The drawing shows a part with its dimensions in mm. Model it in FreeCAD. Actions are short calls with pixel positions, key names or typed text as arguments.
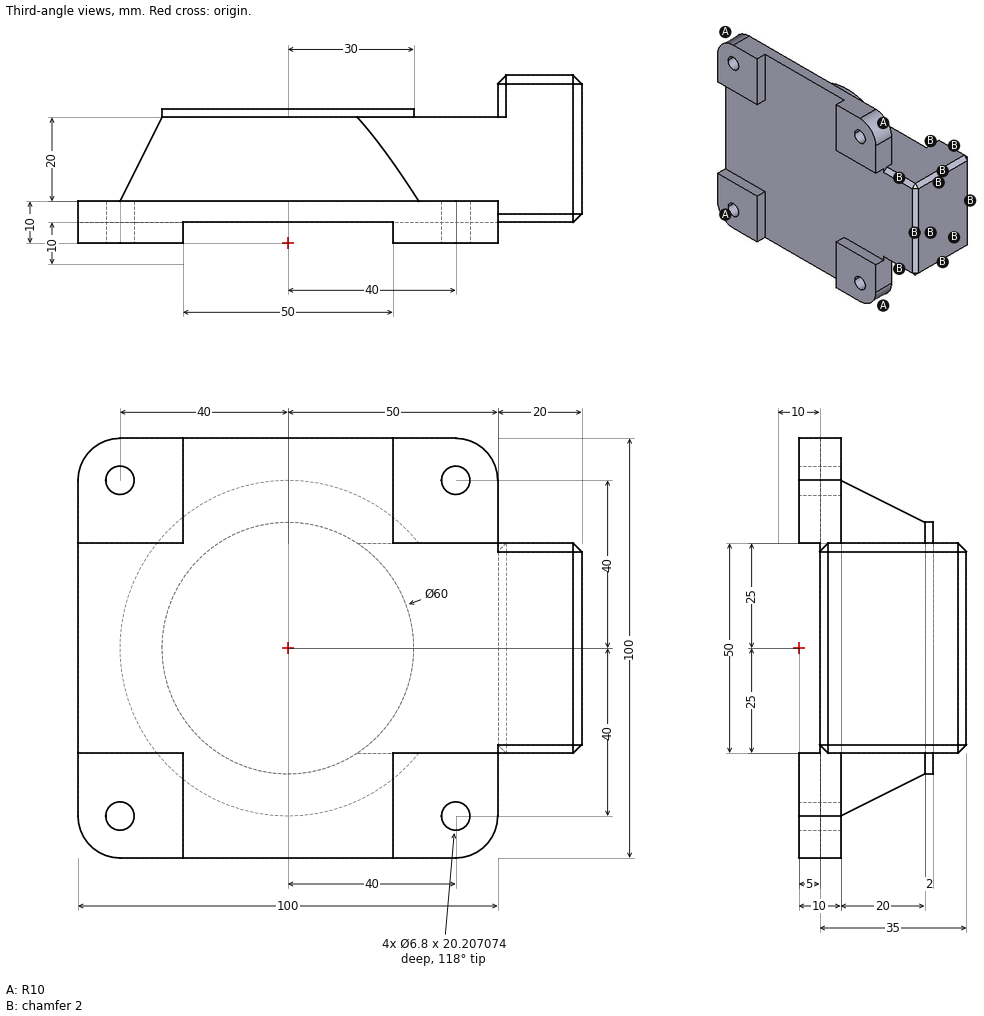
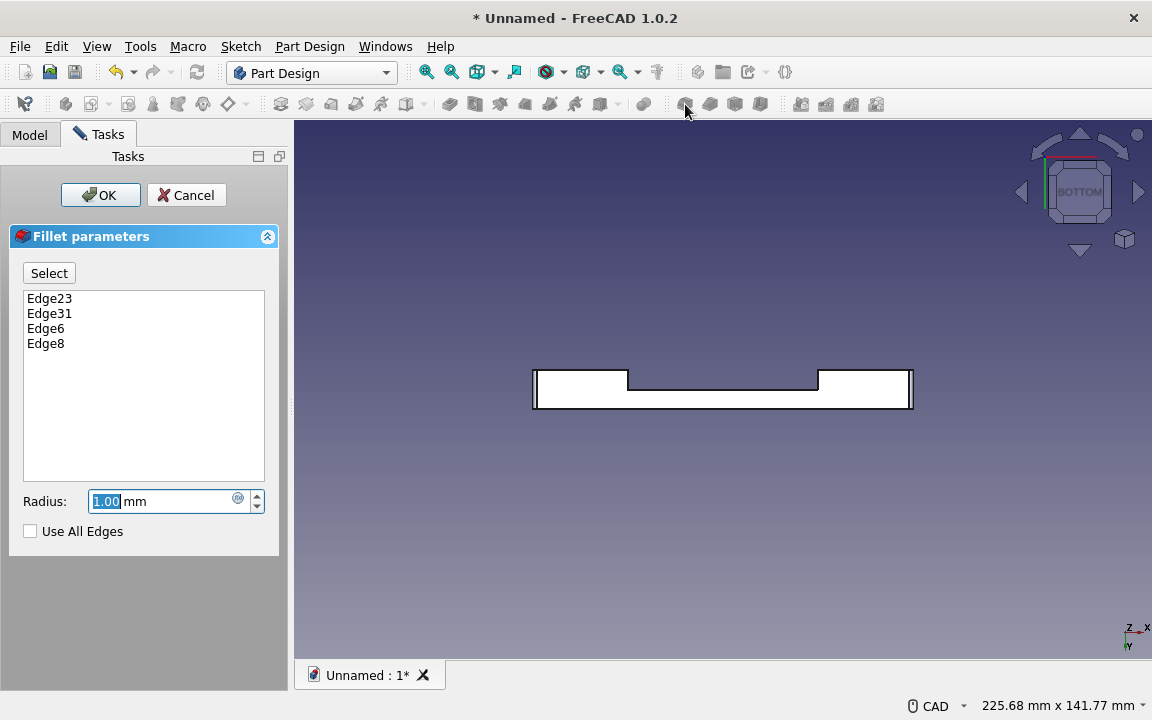
text(10)
key(Tab)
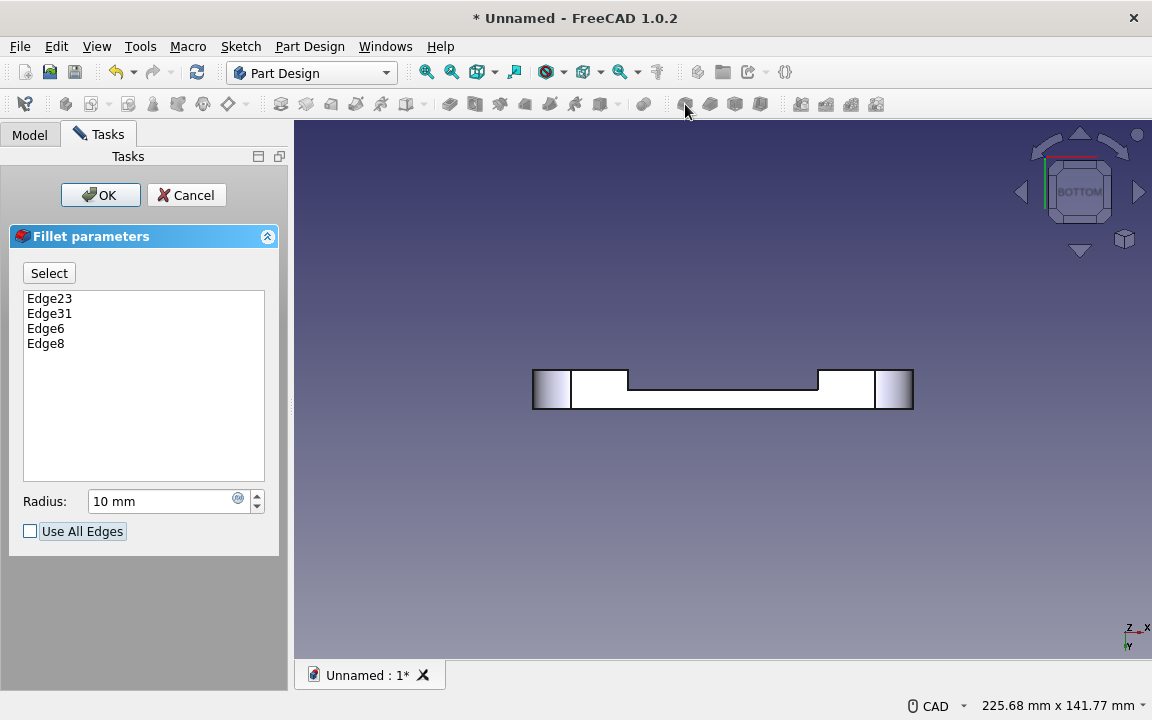
click(101, 195)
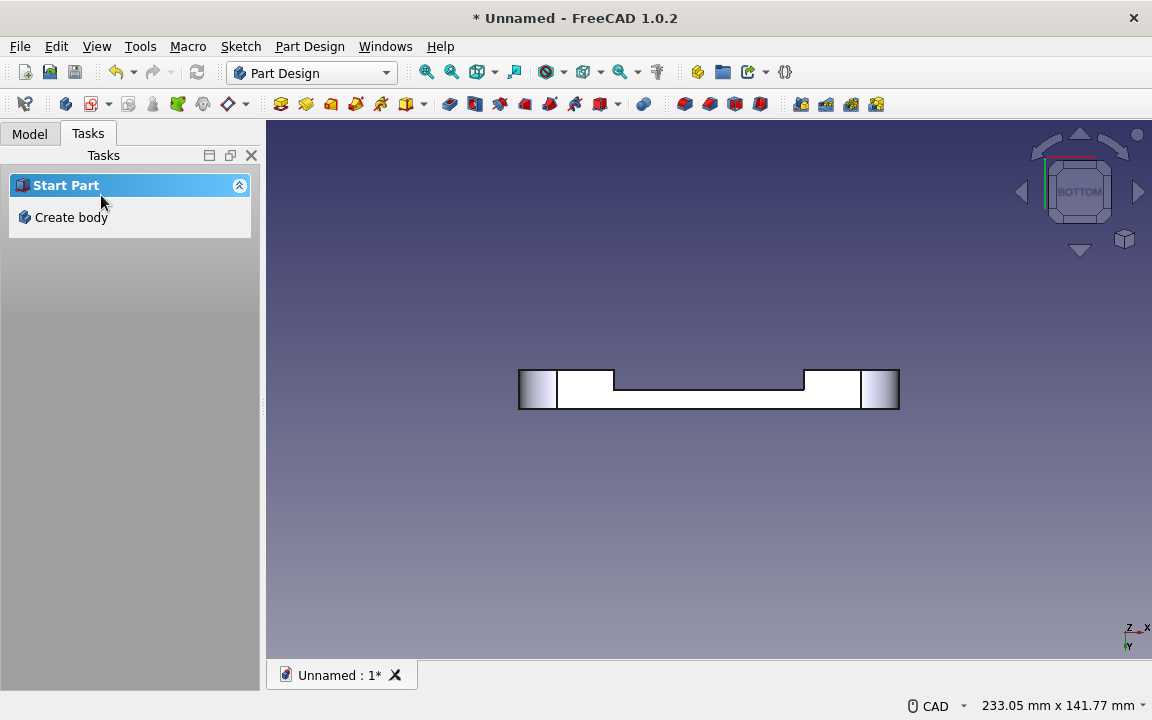
click(427, 72)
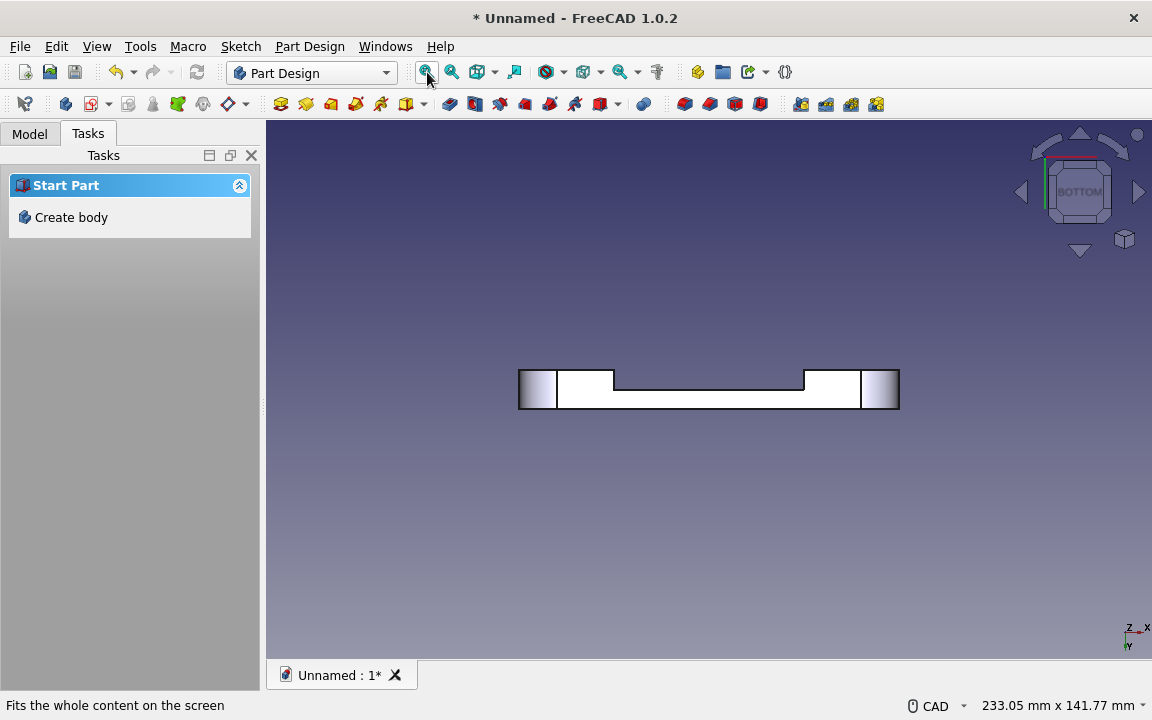
click(90, 104)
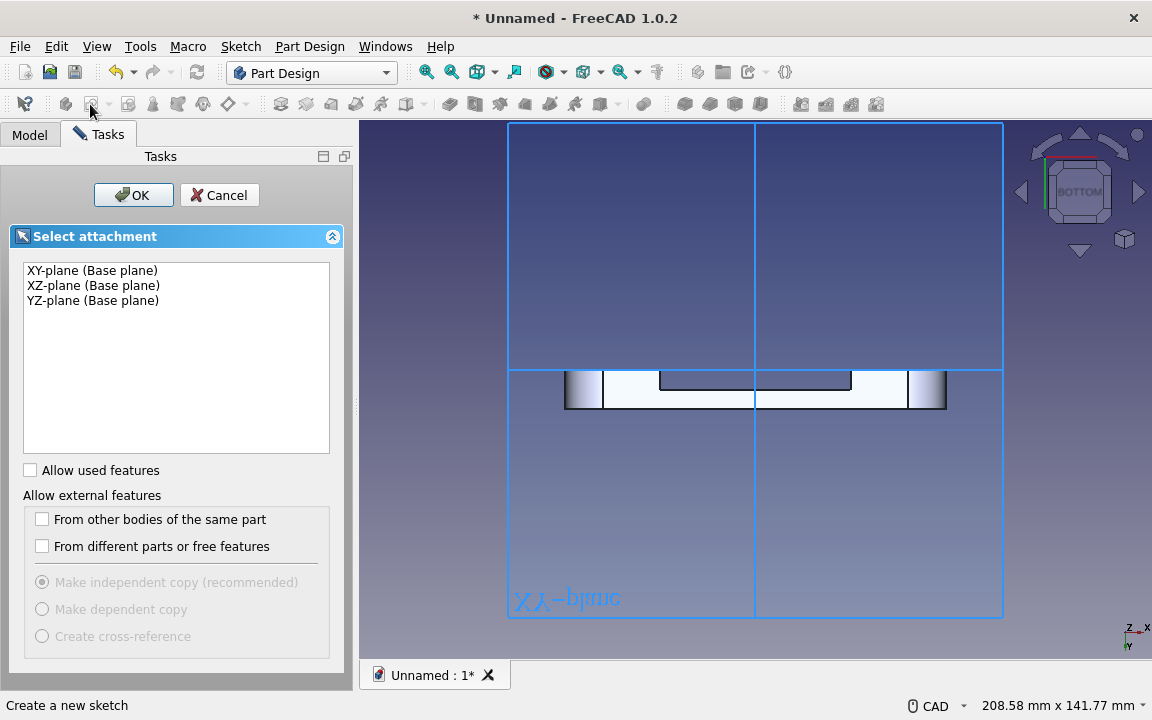
click(84, 270)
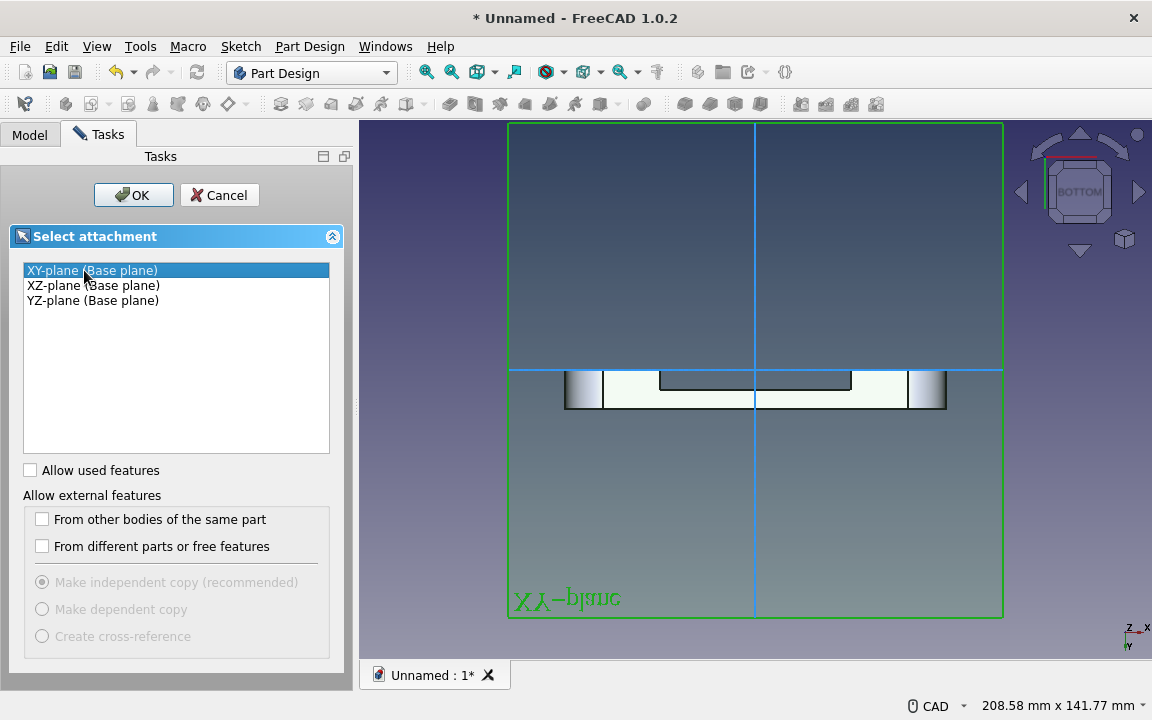
click(134, 195)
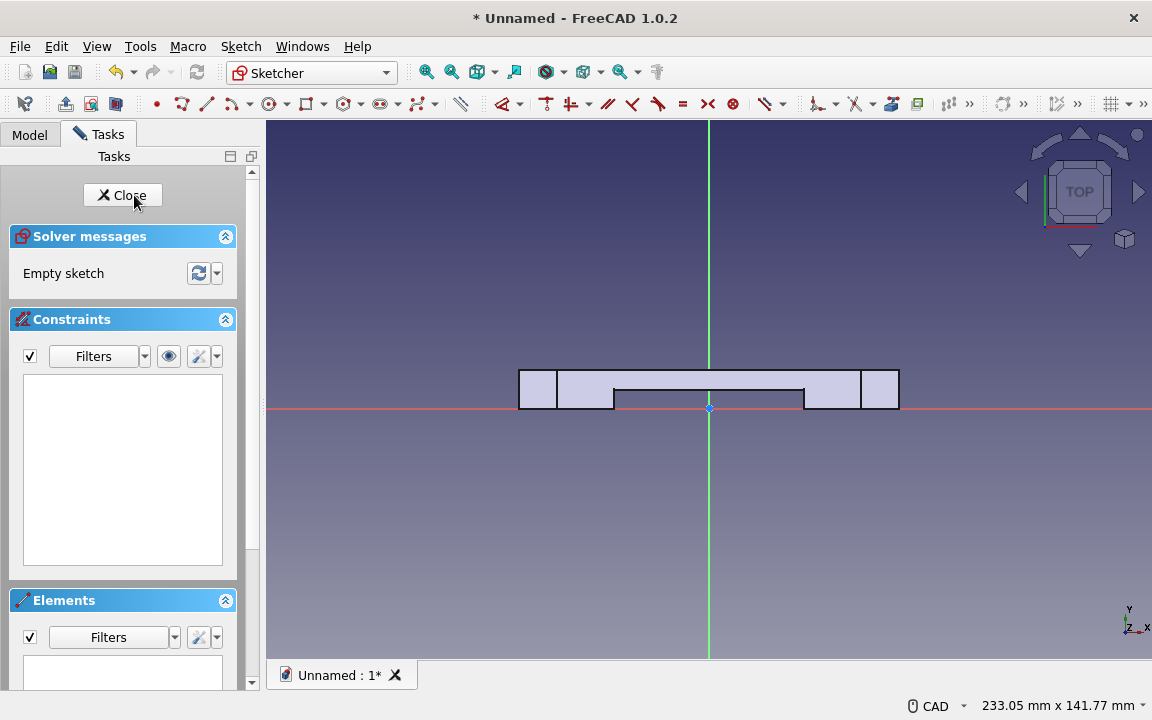
click(116, 104)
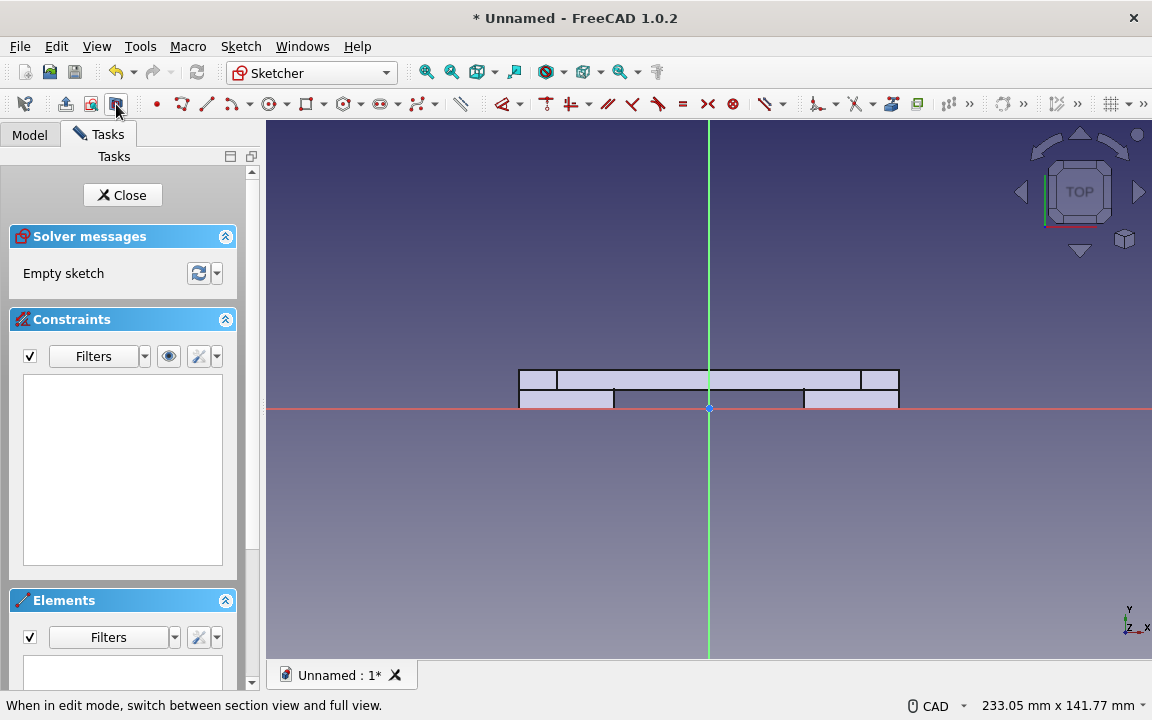
scroll(869, 329, up, 5)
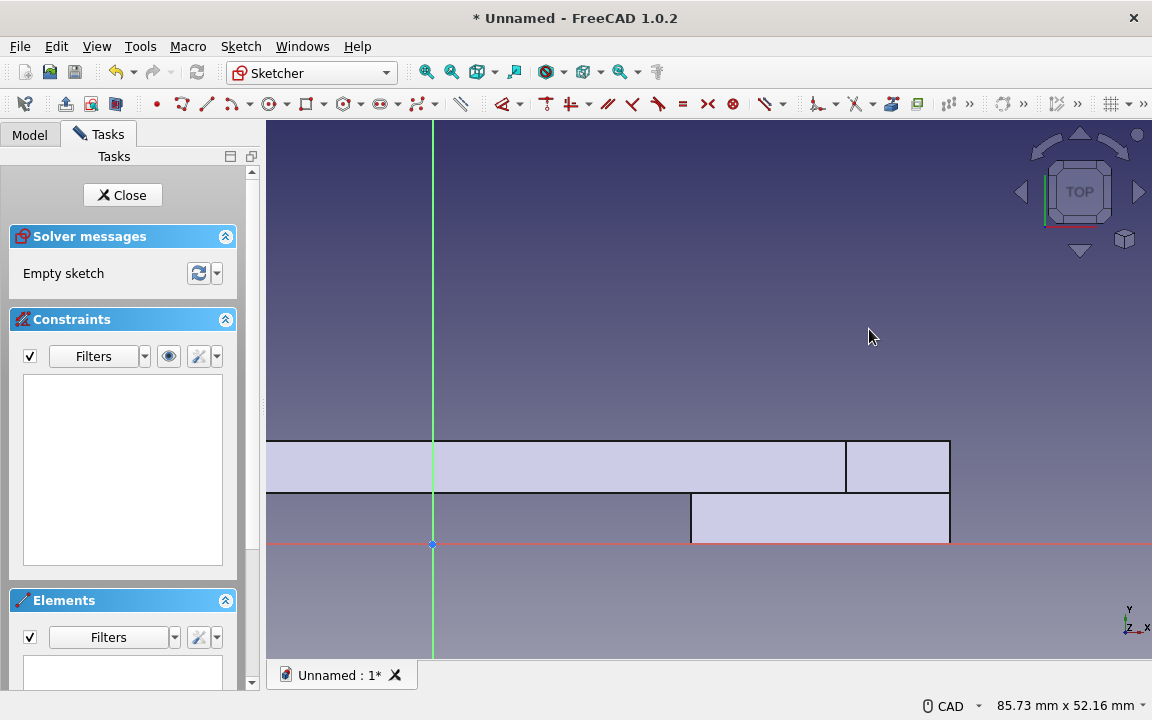
click(182, 104)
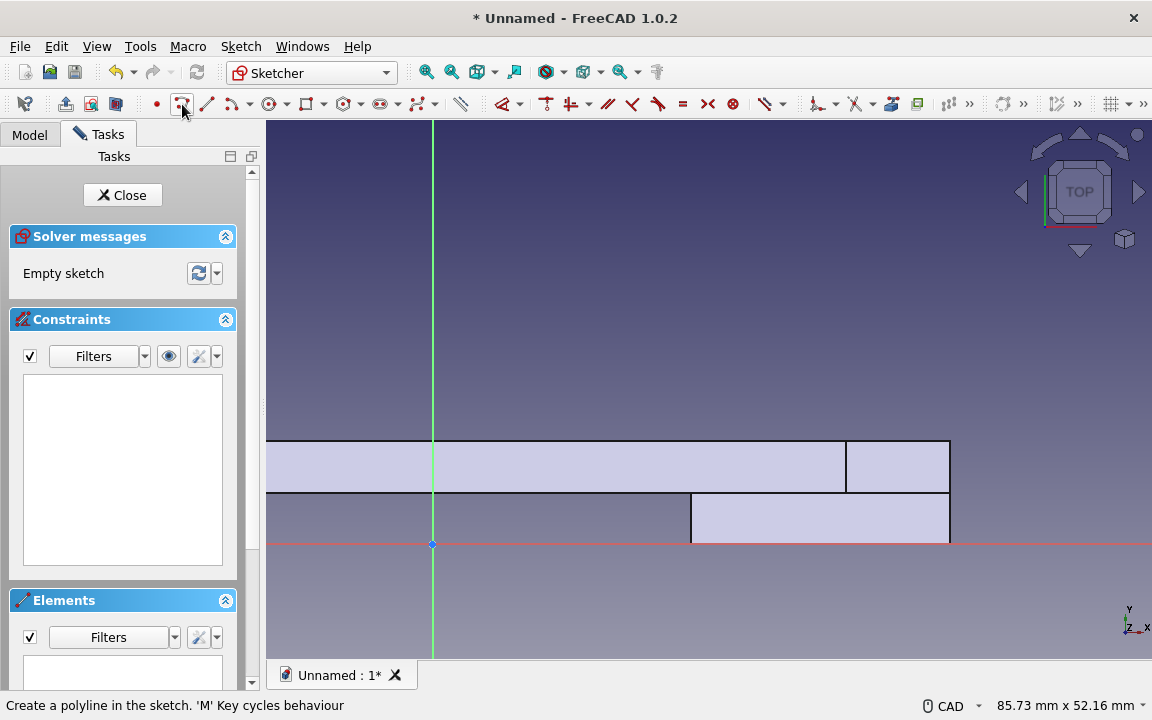
click(433, 441)
click(846, 441)
click(743, 234)
click(442, 234)
click(433, 442)
key(Escape)
key(Escape)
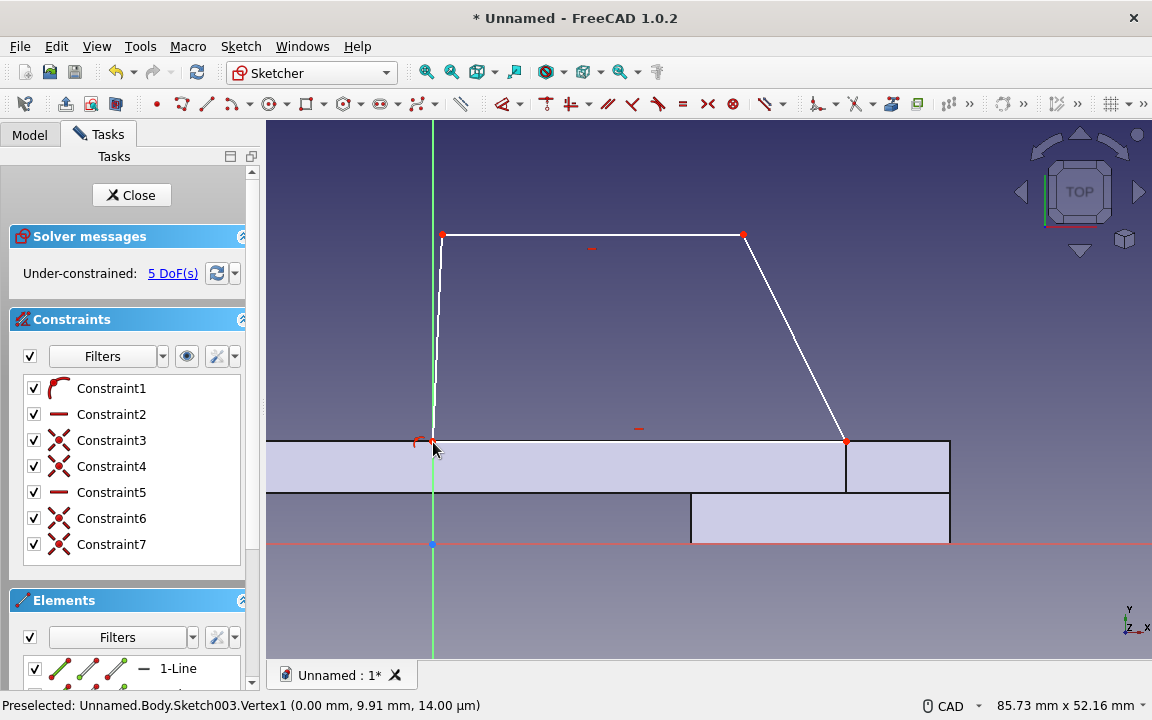
click(436, 380)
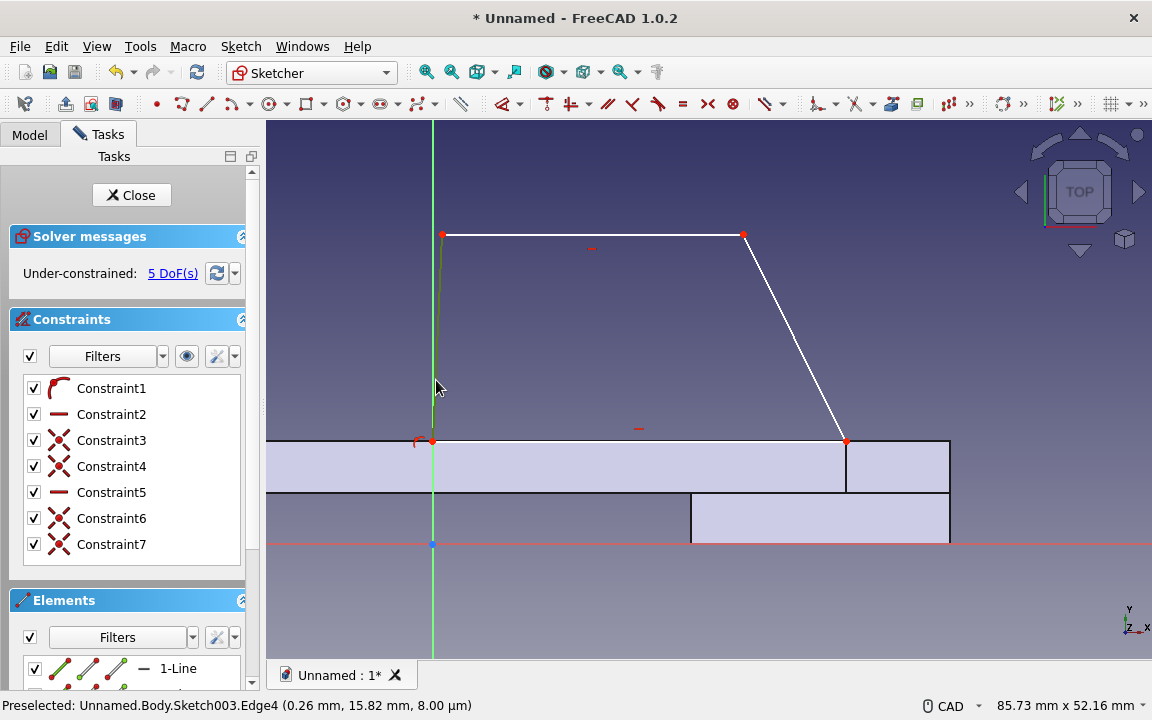
key(v)